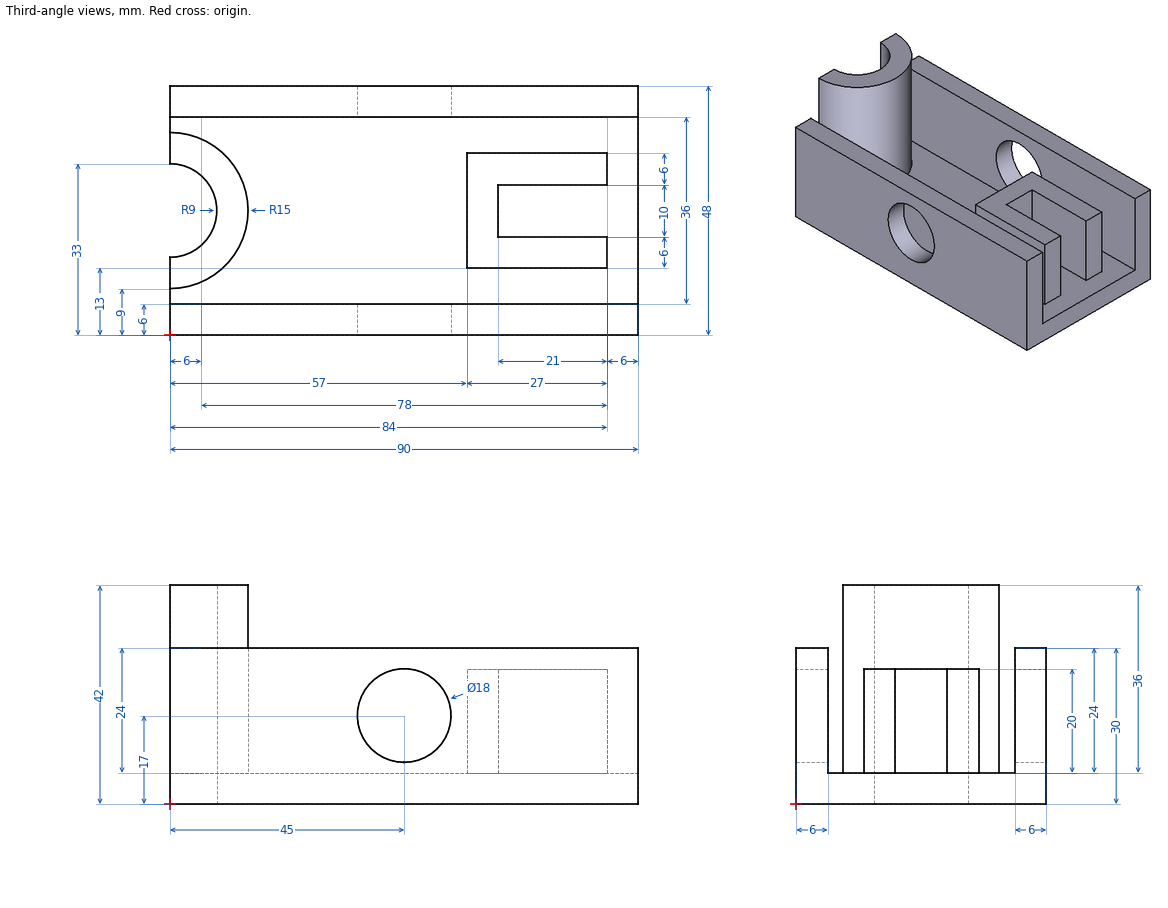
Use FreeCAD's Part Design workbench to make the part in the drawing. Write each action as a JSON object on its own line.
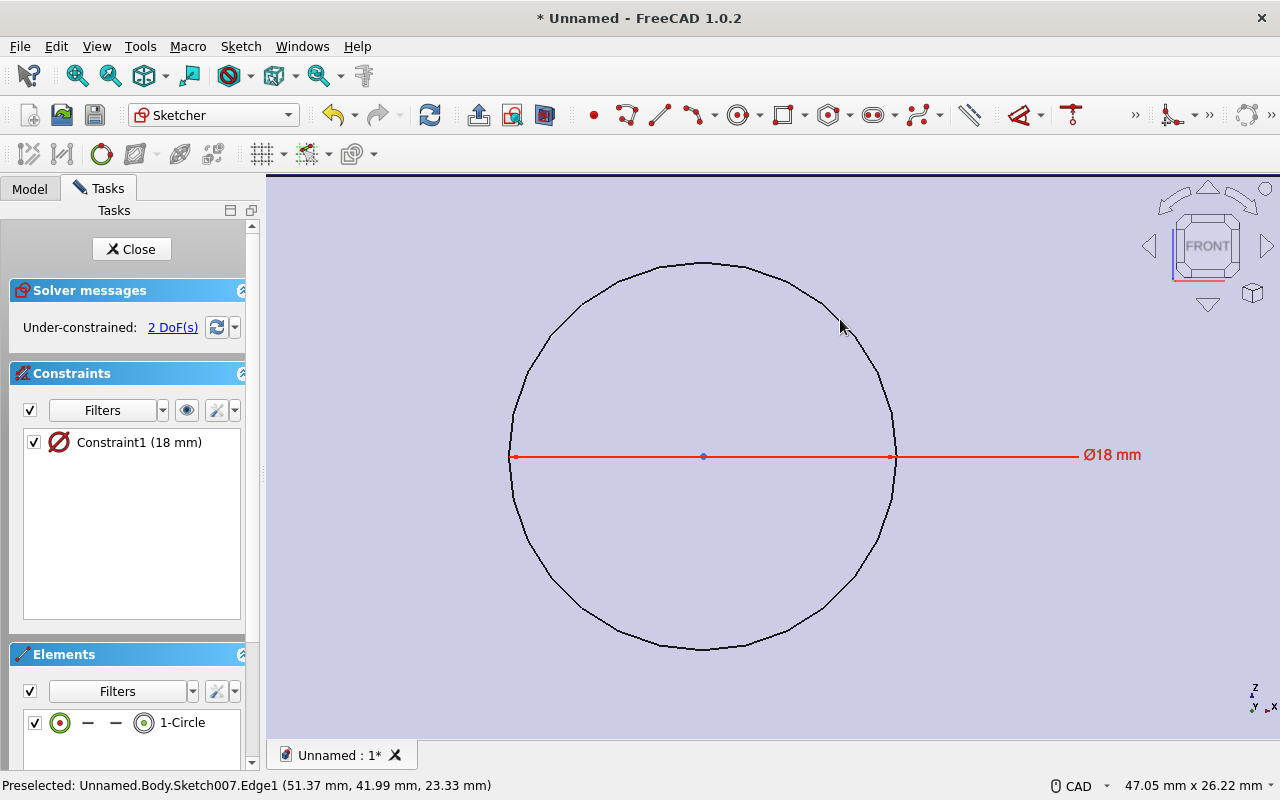
{"action": "left_click", "coordinate": [1018, 116]}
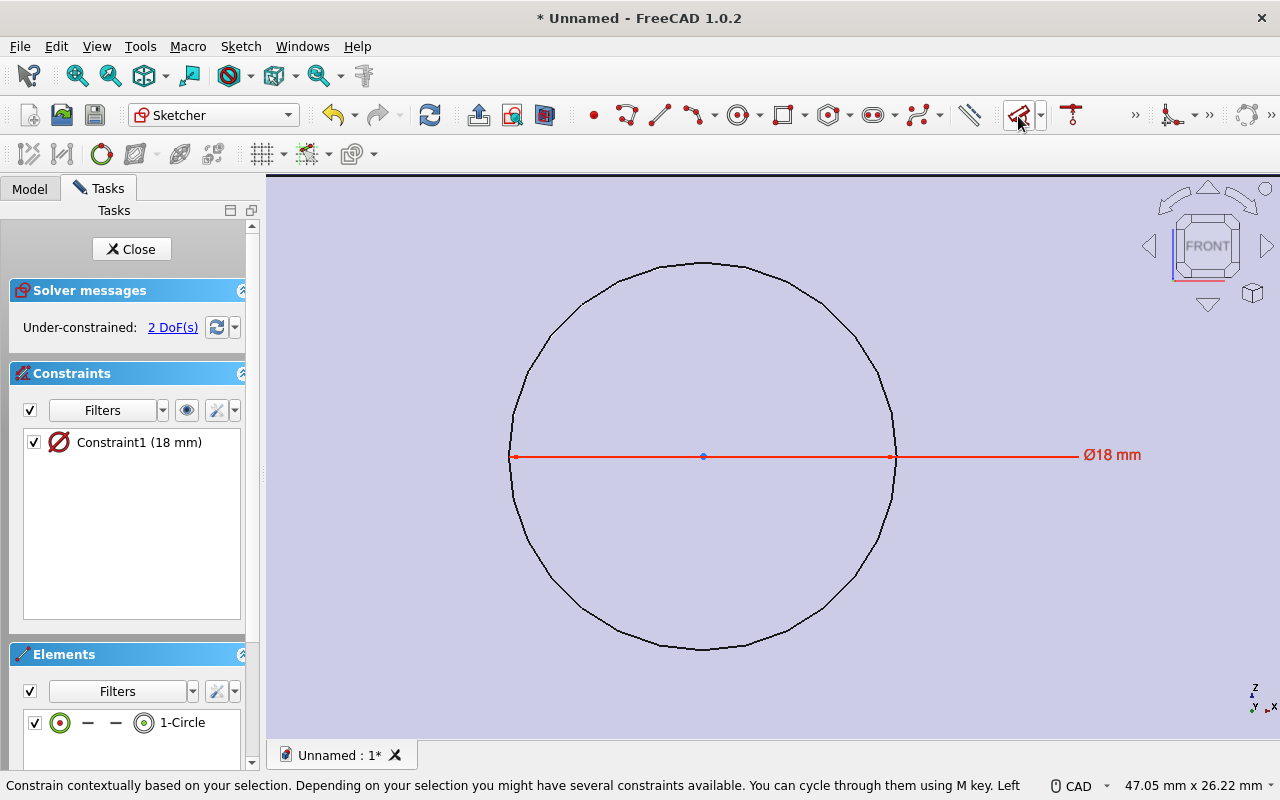
{"action": "left_click", "coordinate": [703, 457]}
{"action": "left_click", "coordinate": [499, 423]}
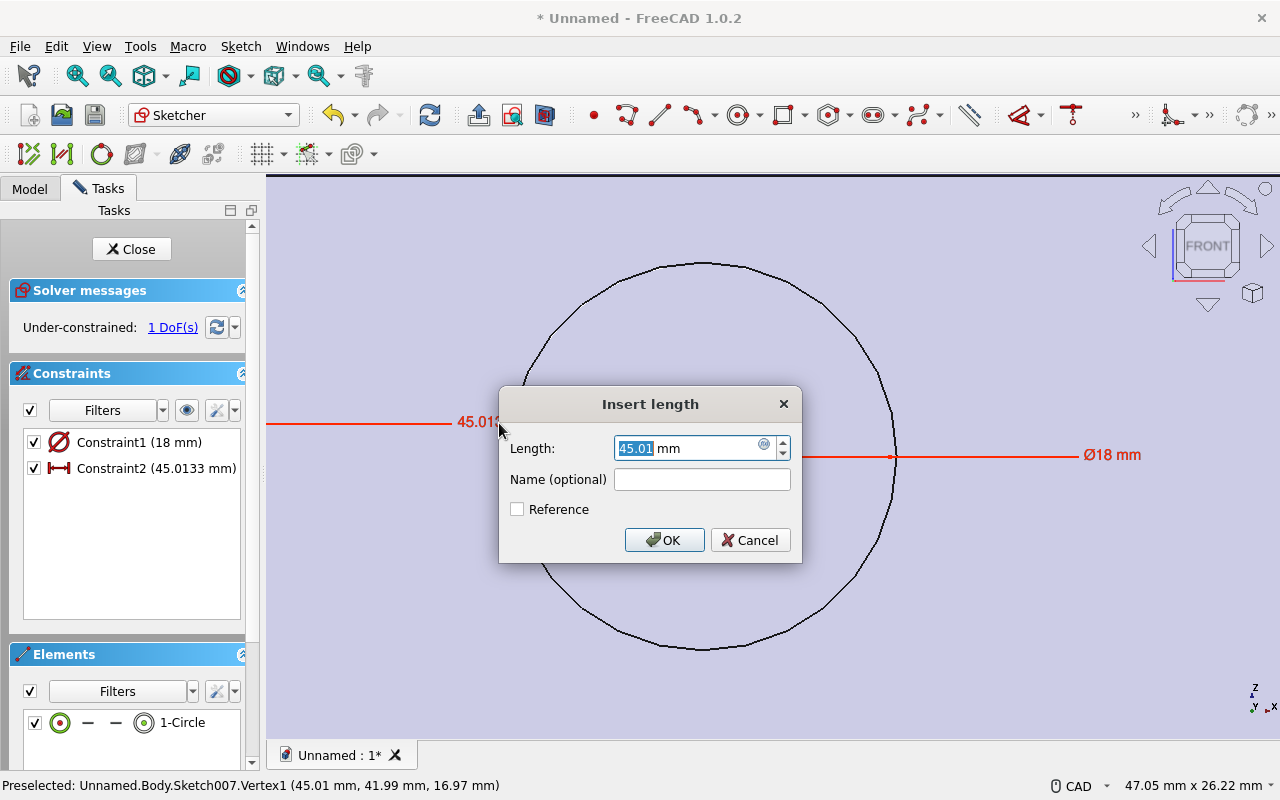
{"action": "type", "text": "45"}
{"action": "key", "text": "Return"}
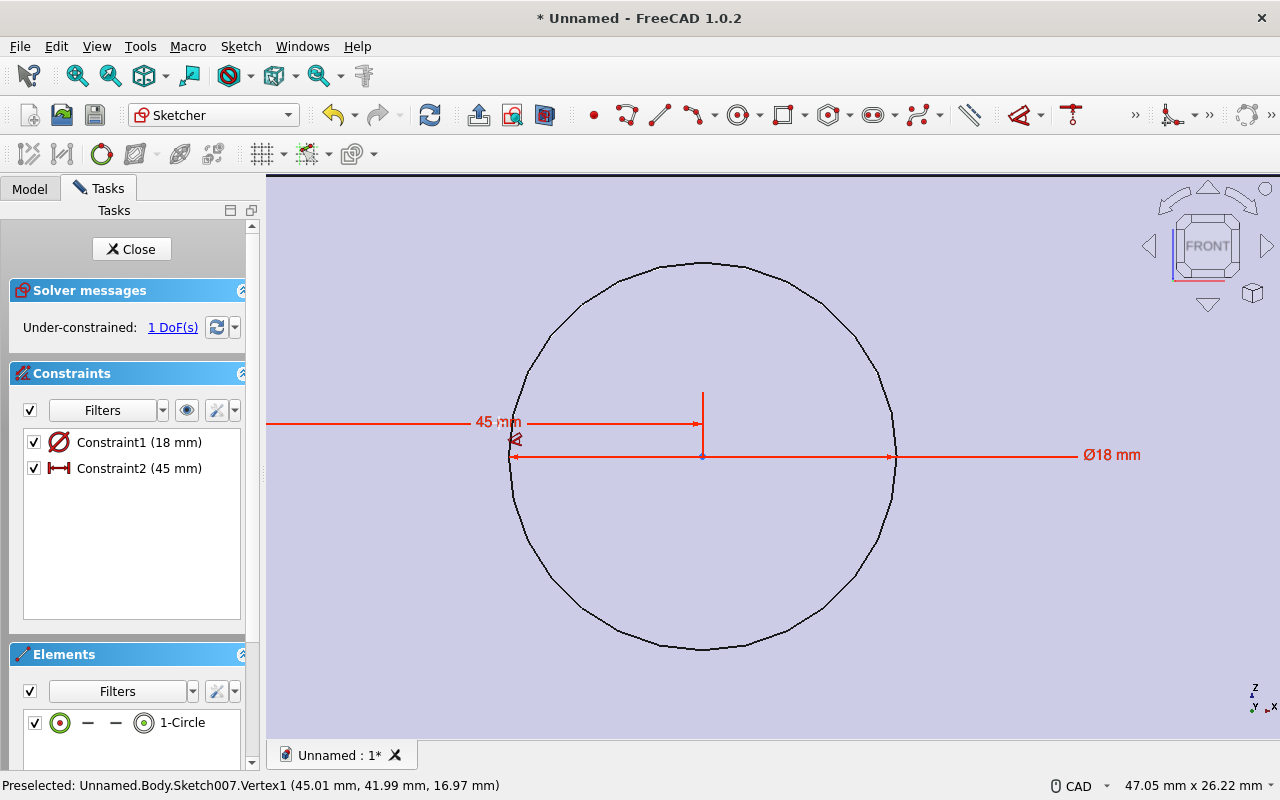
{"action": "left_click", "coordinate": [703, 457]}
{"action": "left_click", "coordinate": [737, 584]}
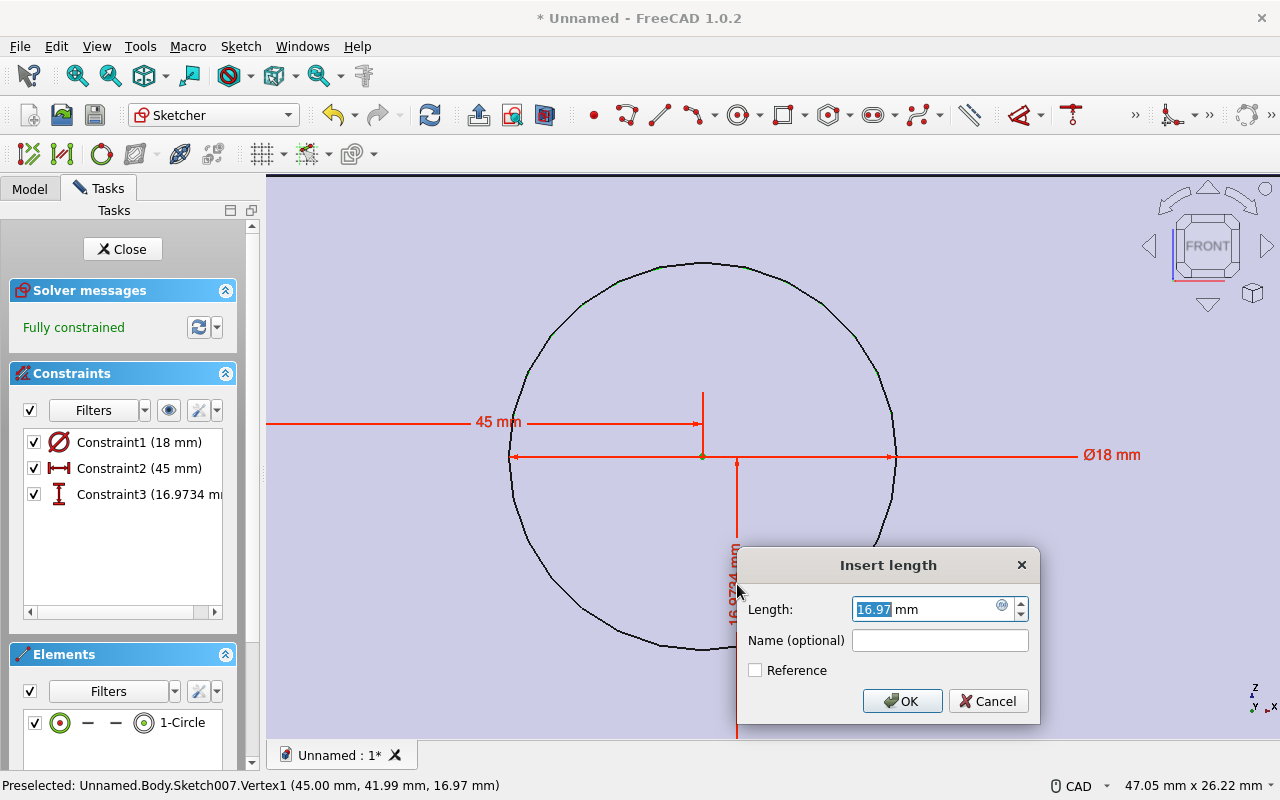
{"action": "type", "text": "17"}
{"action": "key", "text": "Return"}
{"action": "key", "text": "Escape"}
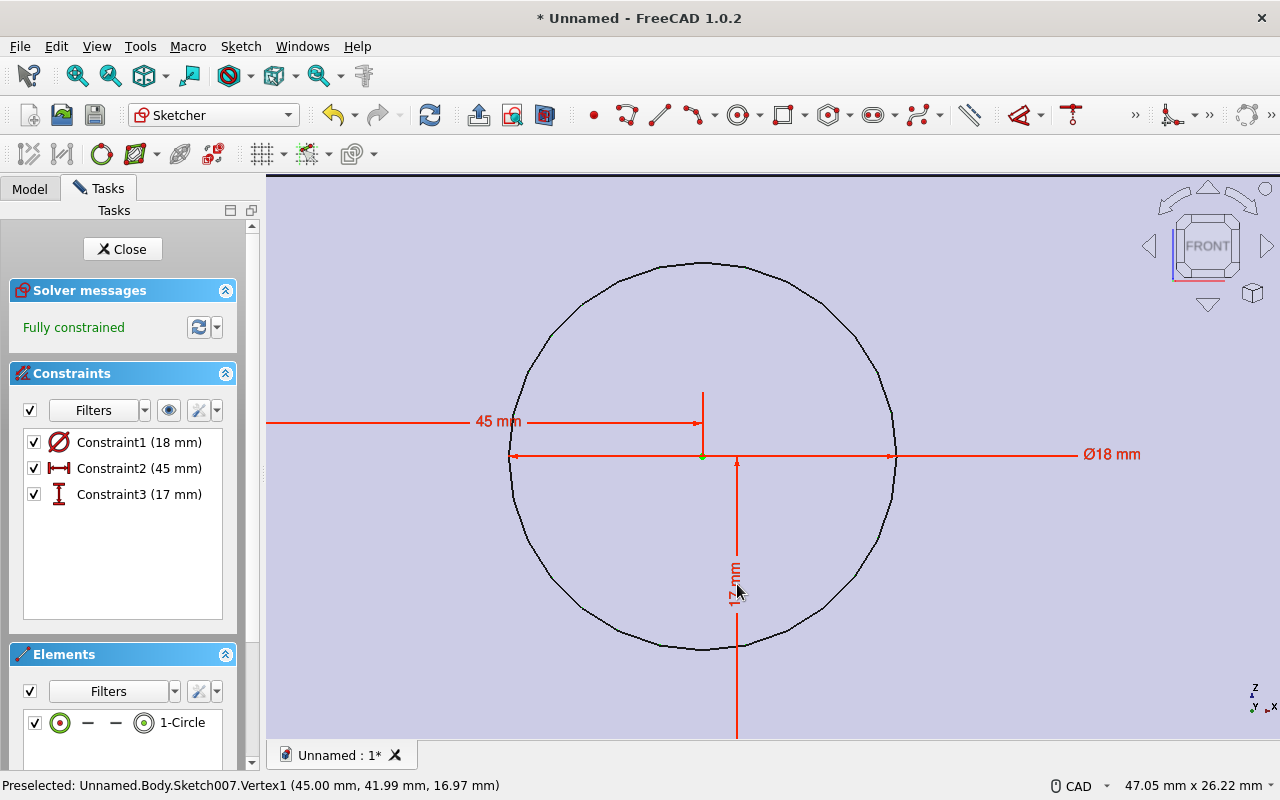
{"action": "left_click", "coordinate": [123, 249]}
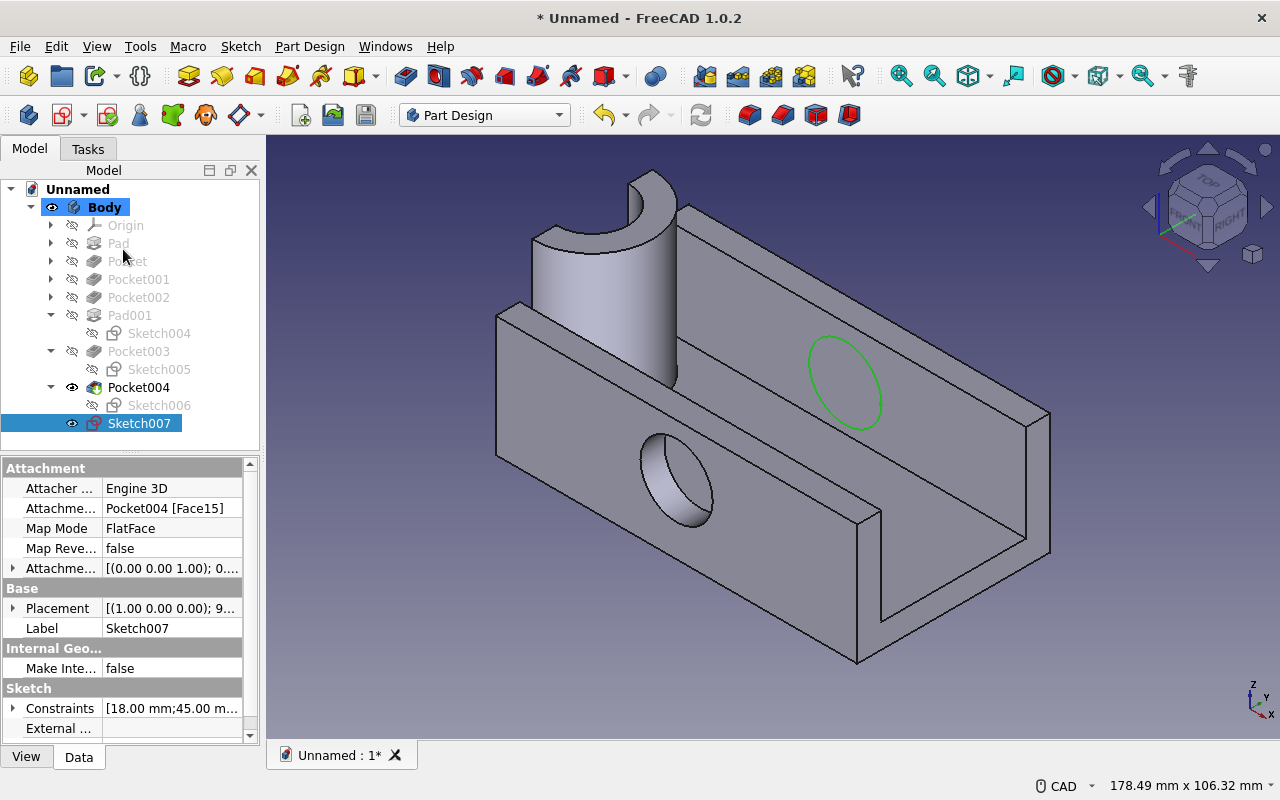
{"action": "left_click", "coordinate": [406, 76]}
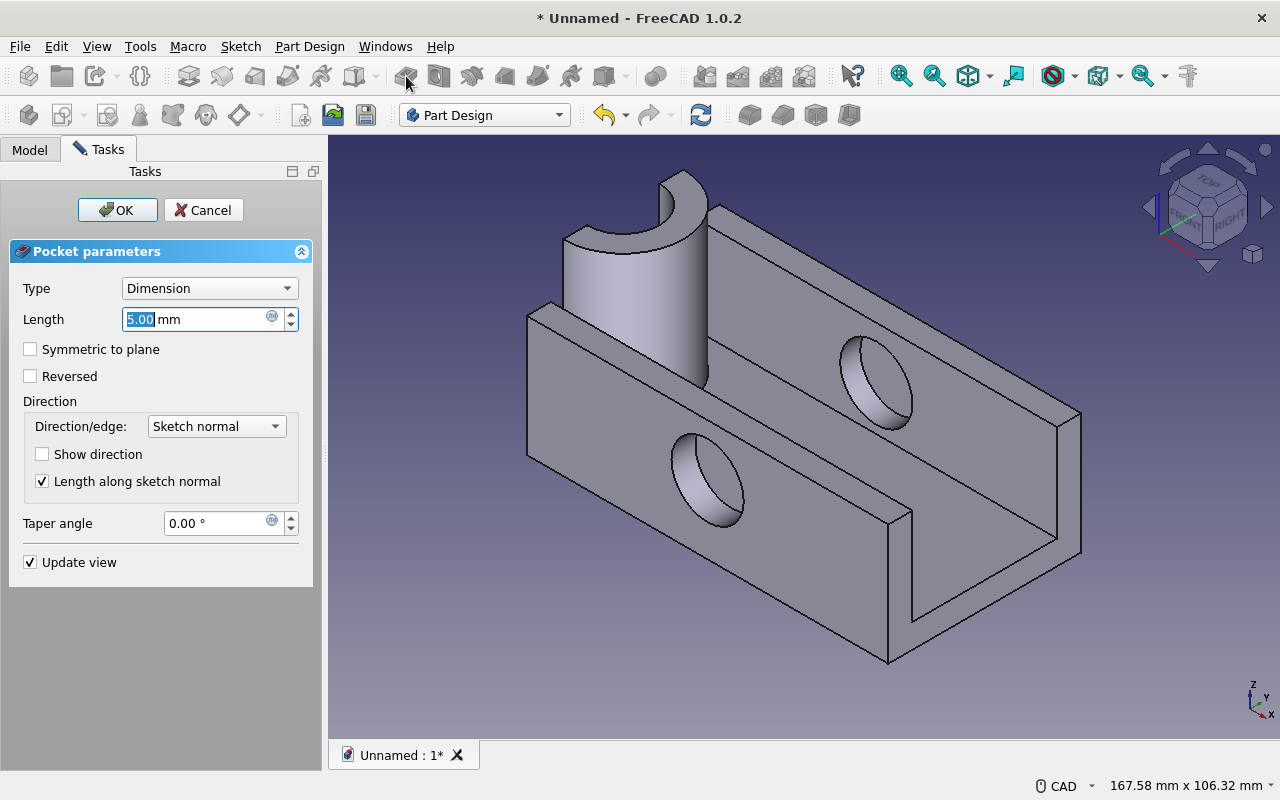
{"action": "type", "text": "6"}
{"action": "key", "text": "Tab"}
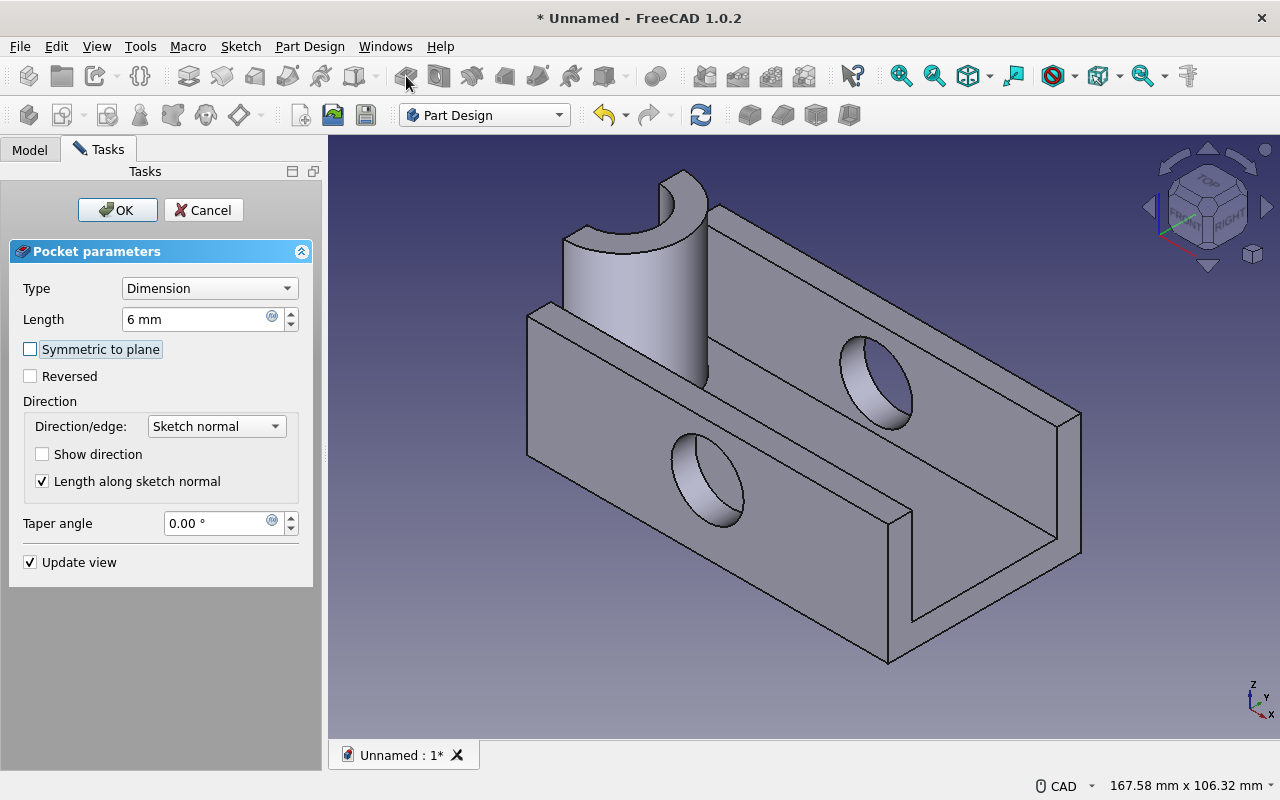
{"action": "left_click", "coordinate": [118, 210]}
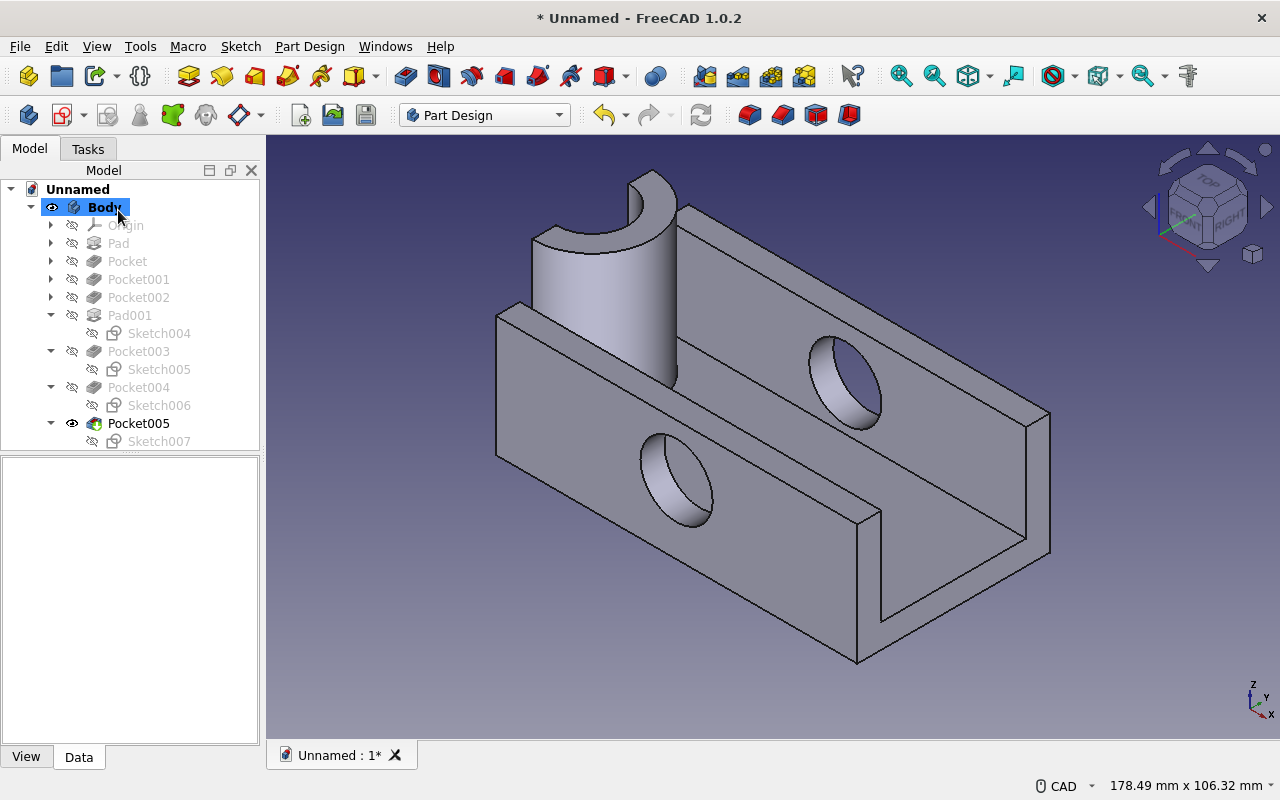
{"action": "left_click", "coordinate": [897, 523]}